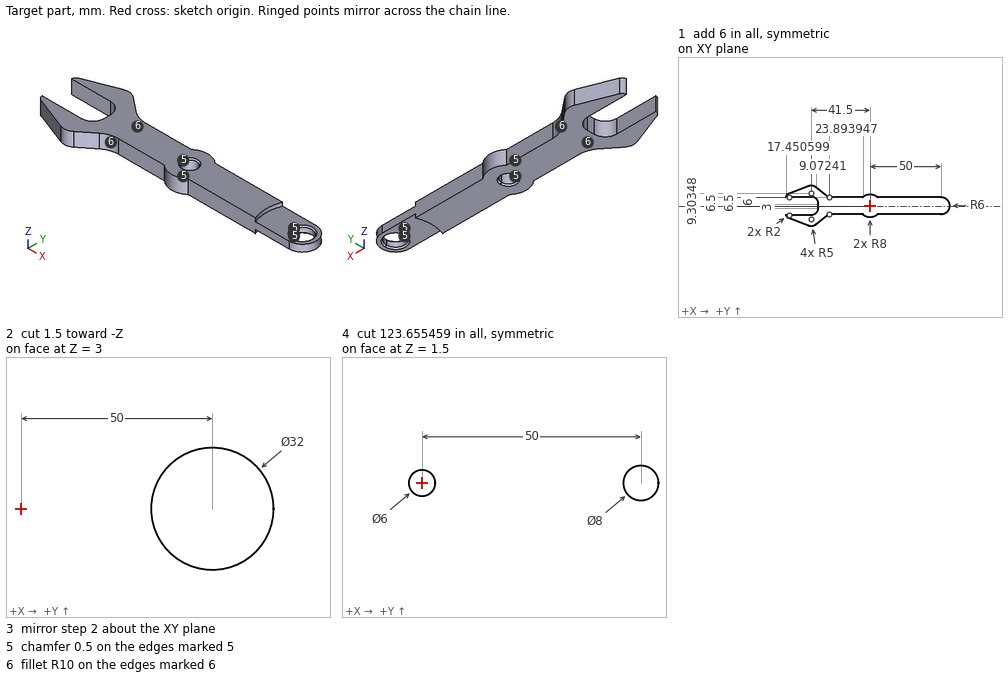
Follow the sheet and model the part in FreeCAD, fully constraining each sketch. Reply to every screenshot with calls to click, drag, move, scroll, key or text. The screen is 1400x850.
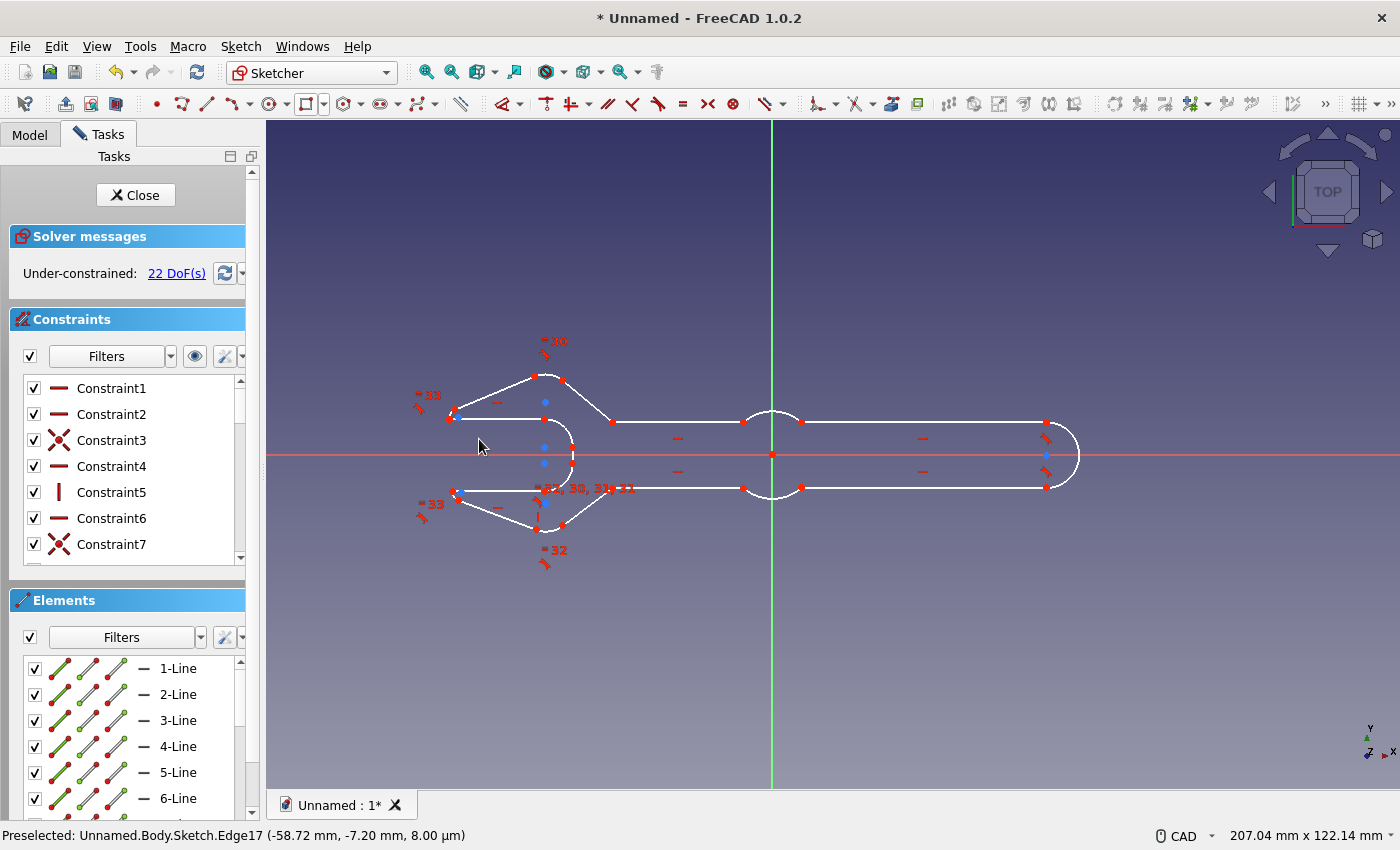
click(785, 413)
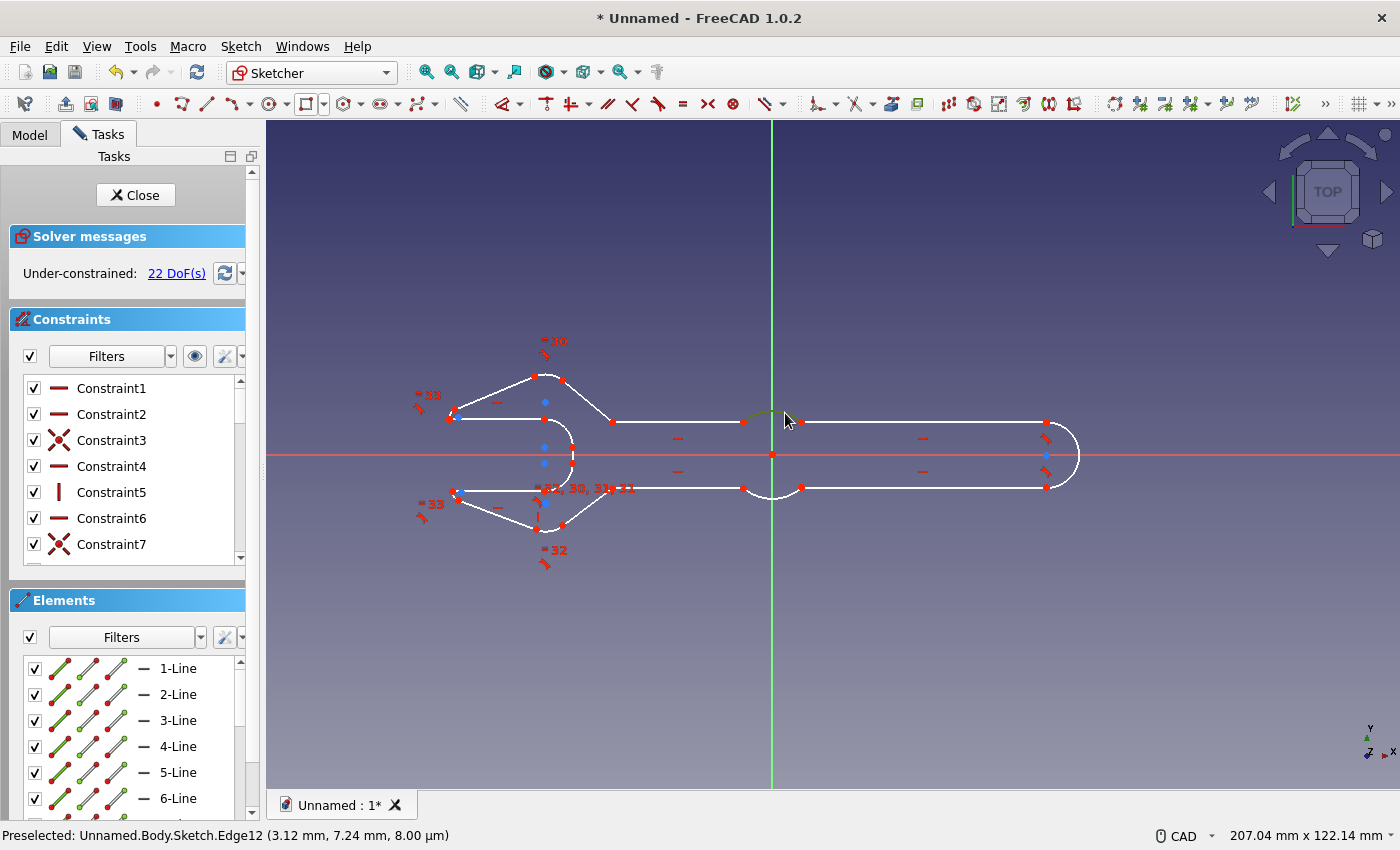
click(760, 497)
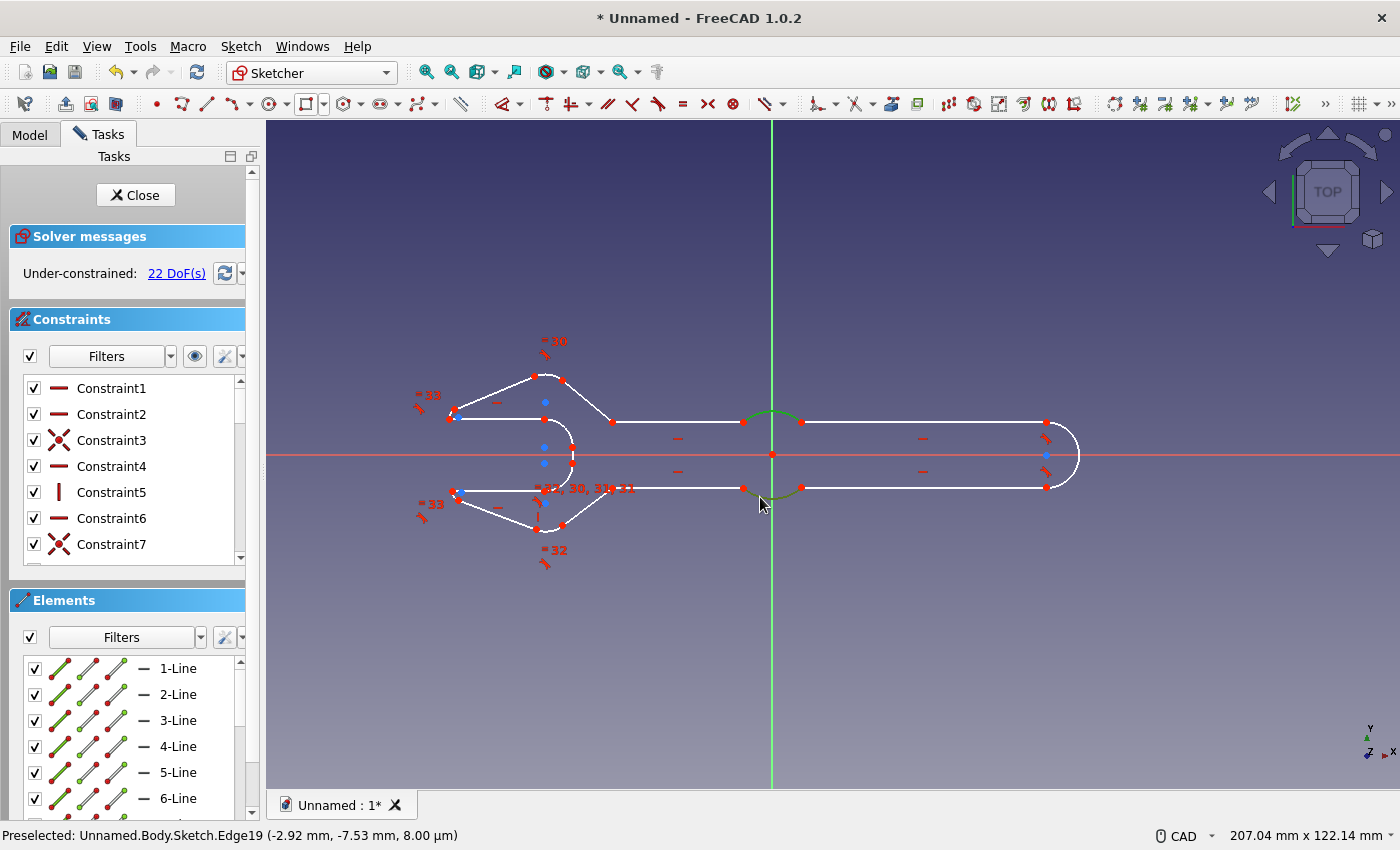
click(683, 104)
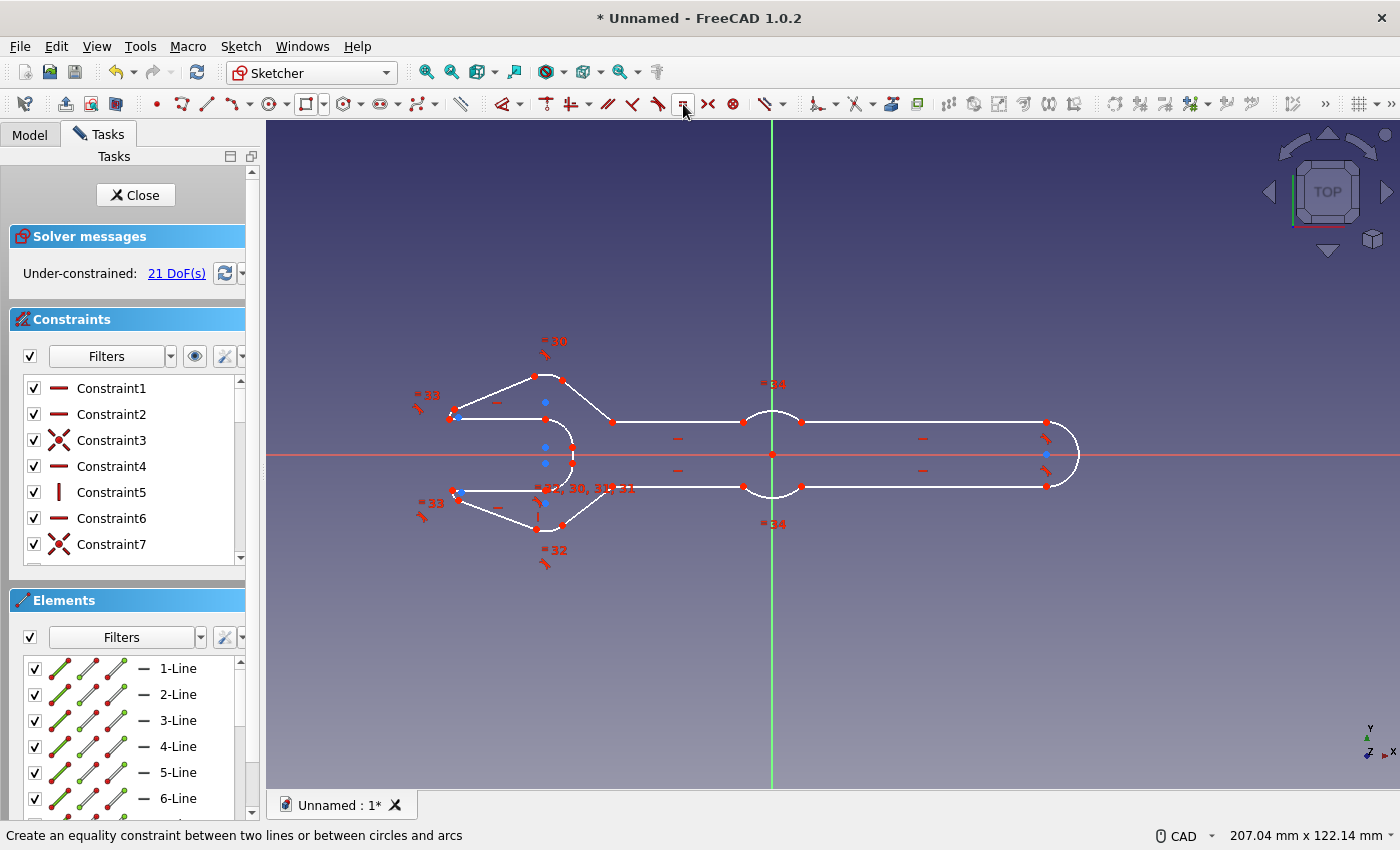
click(1046, 454)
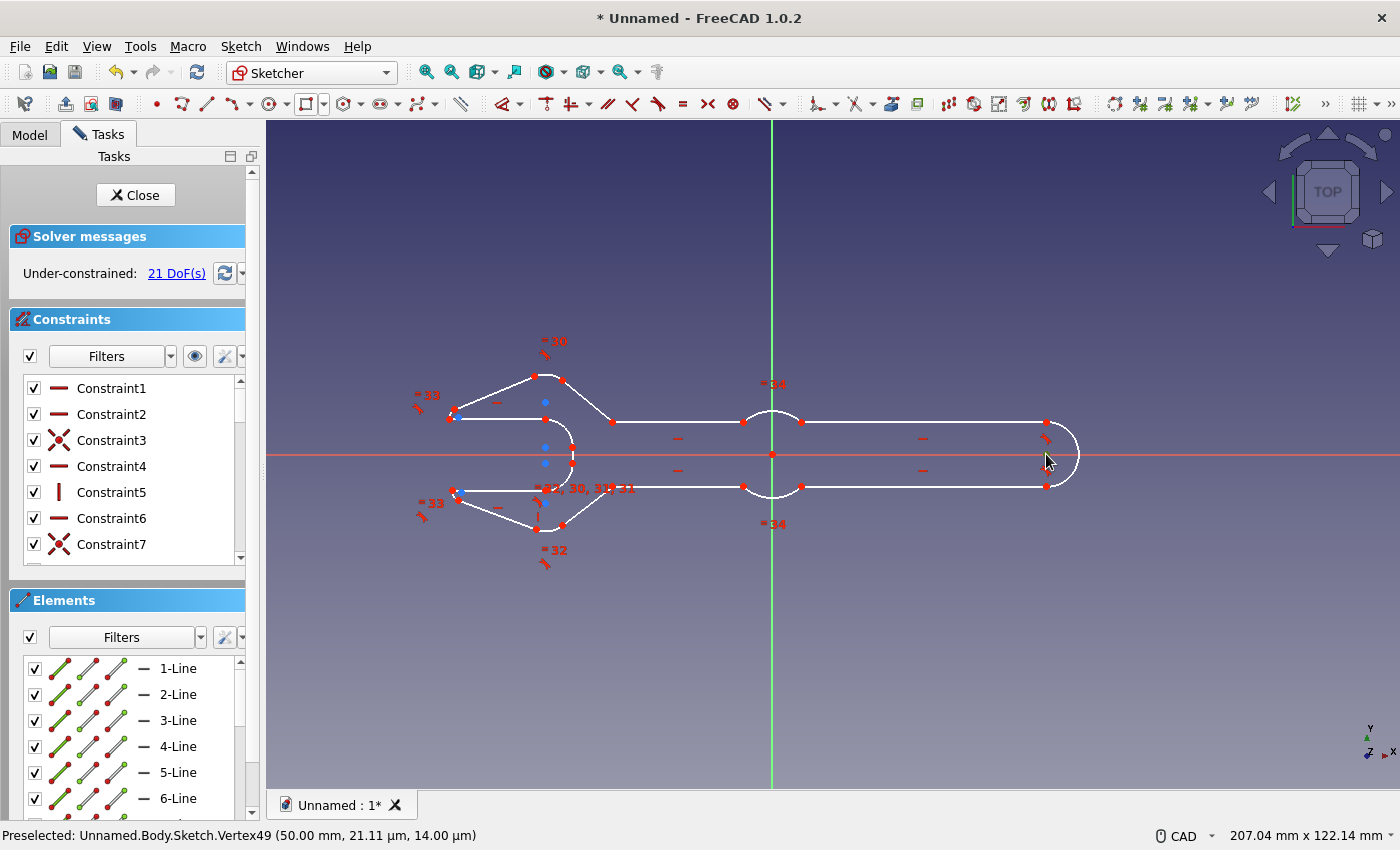
click(361, 455)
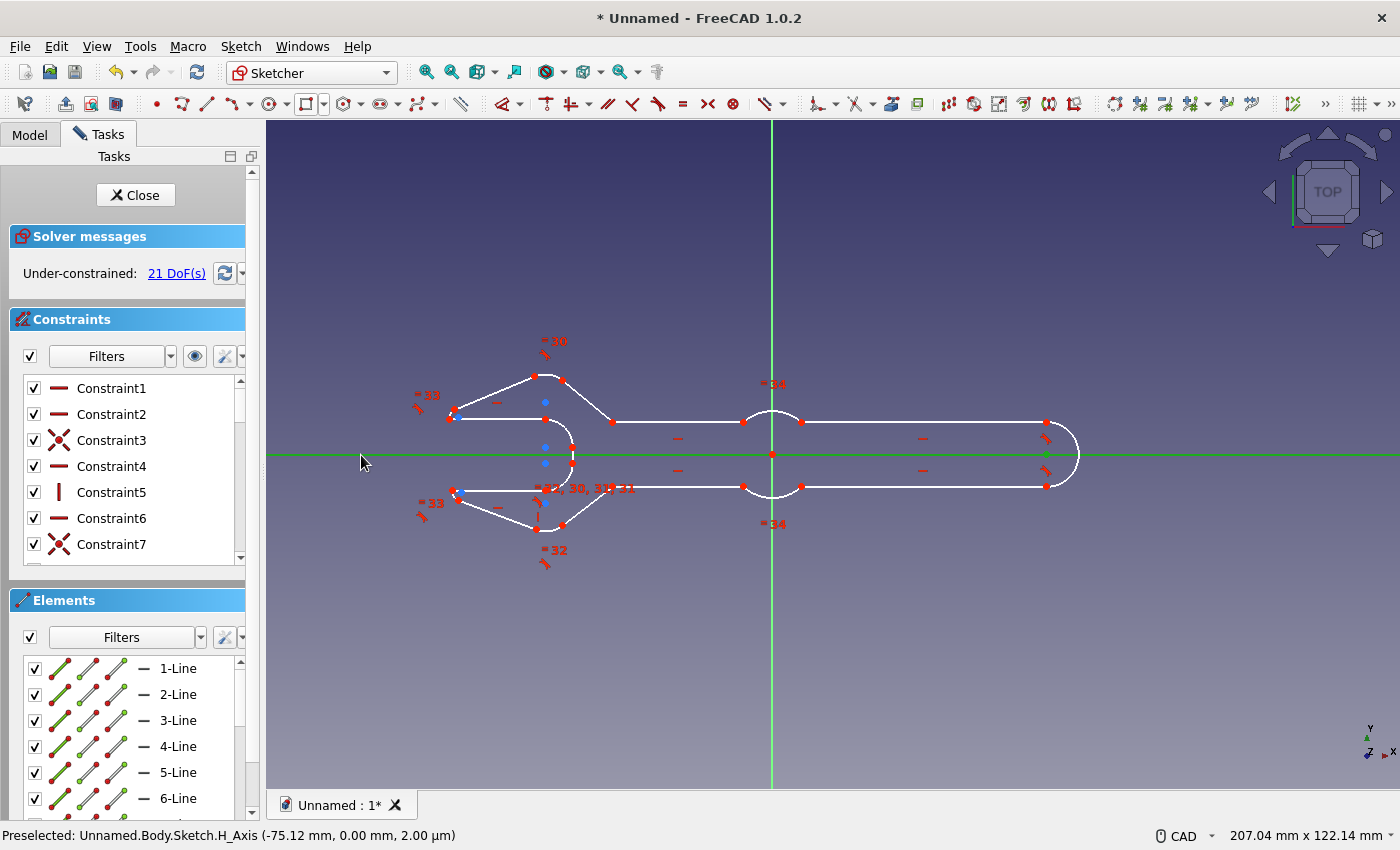
click(546, 104)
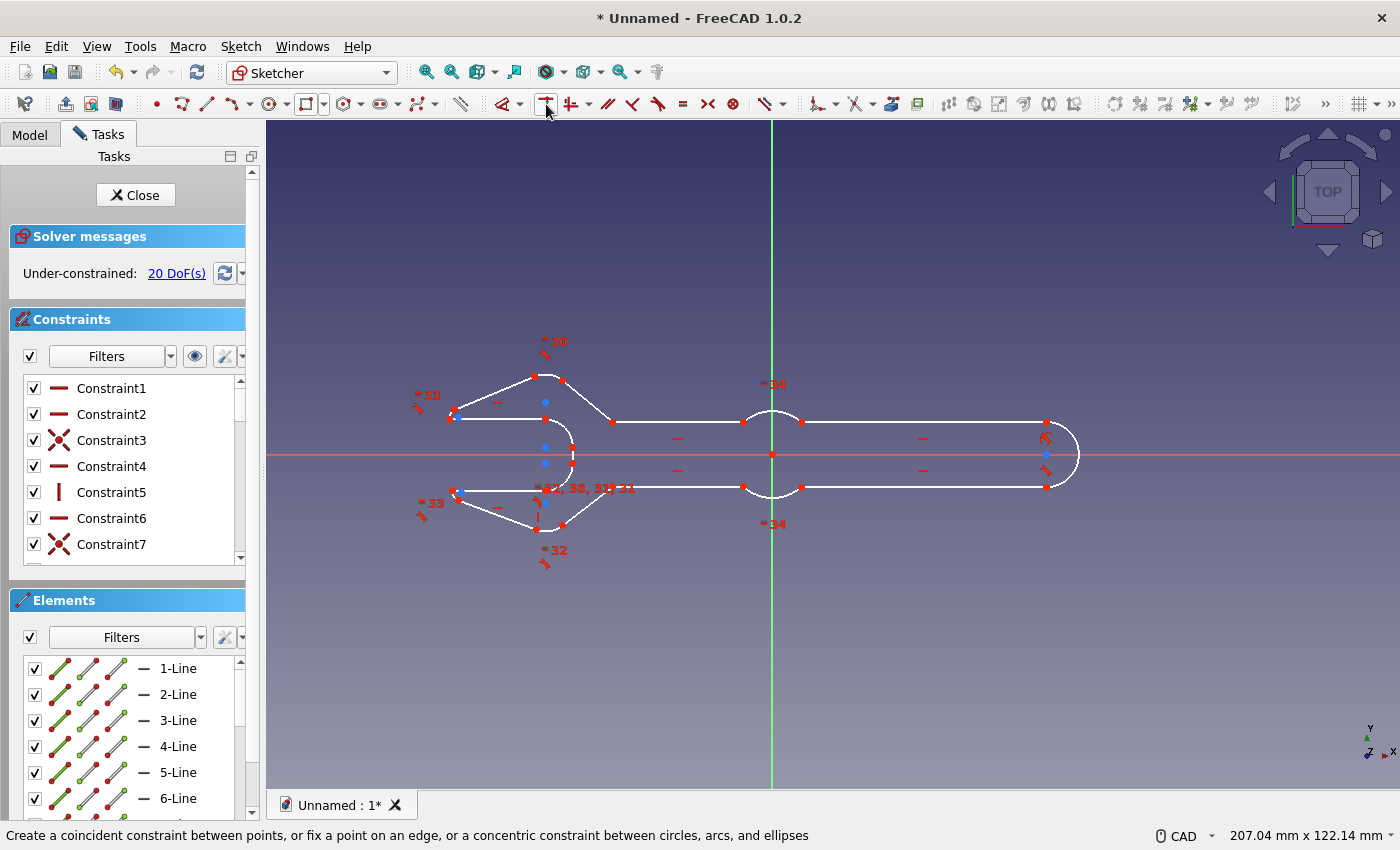
scroll(458, 418, up, 2)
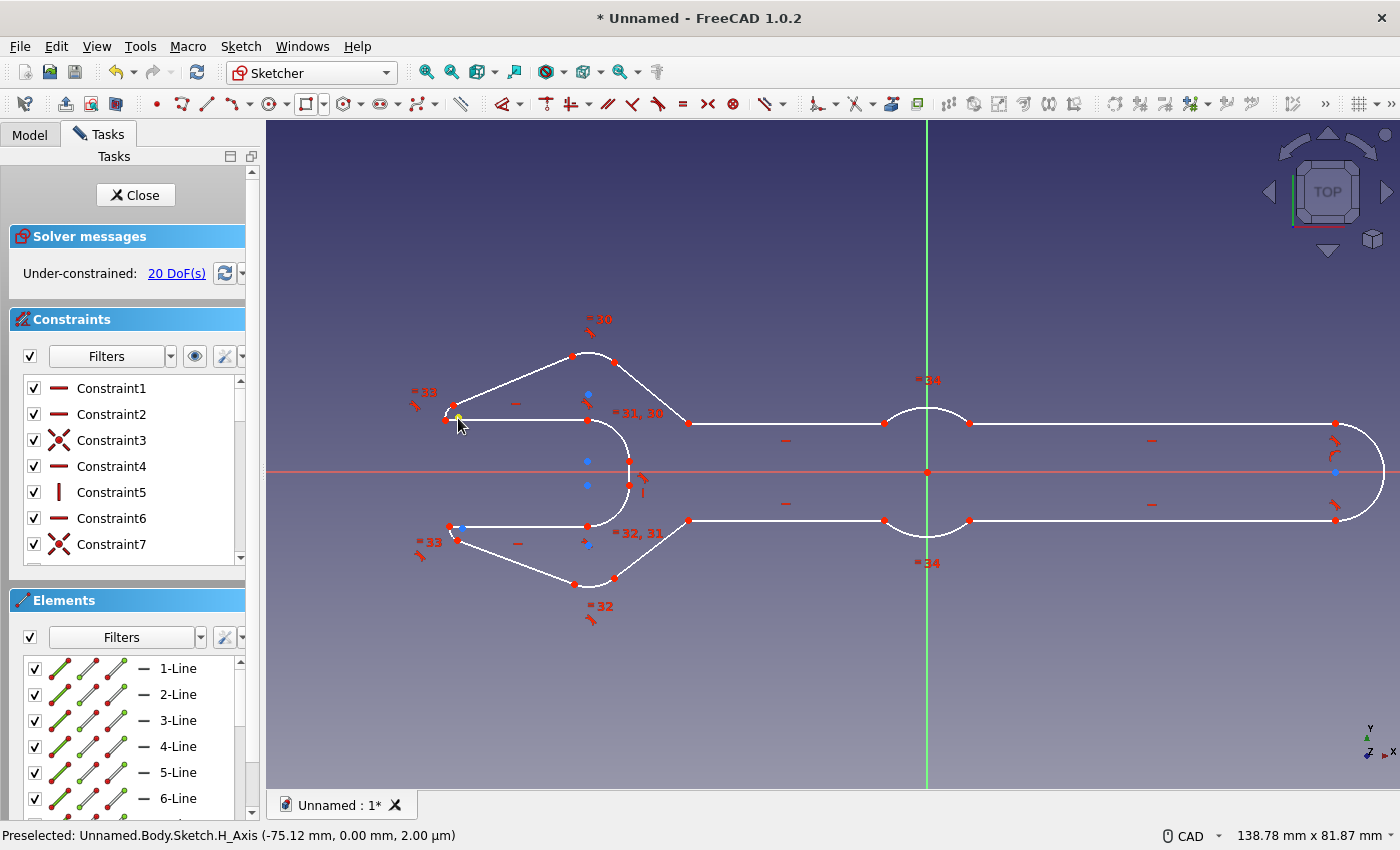
click(458, 417)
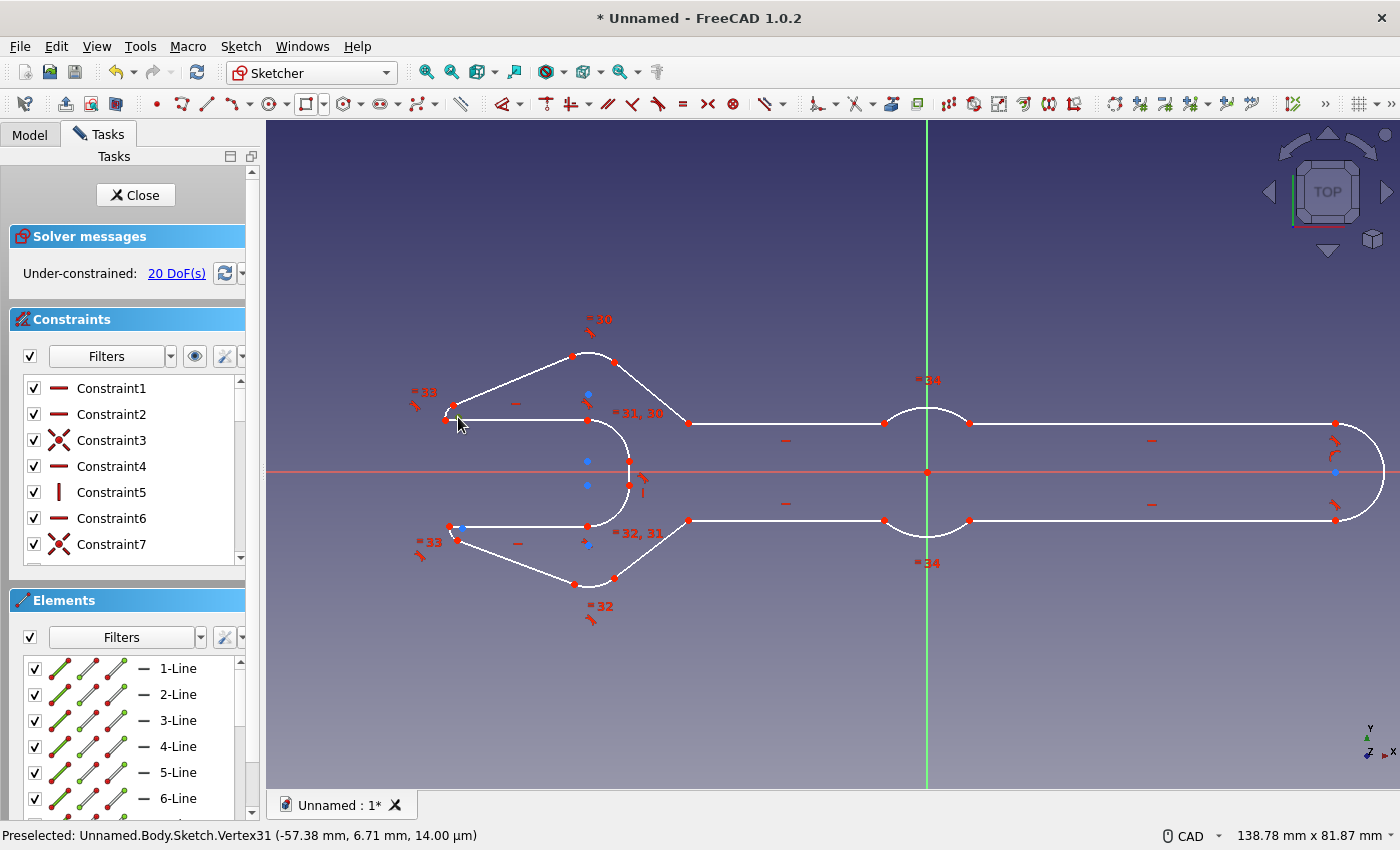
click(462, 529)